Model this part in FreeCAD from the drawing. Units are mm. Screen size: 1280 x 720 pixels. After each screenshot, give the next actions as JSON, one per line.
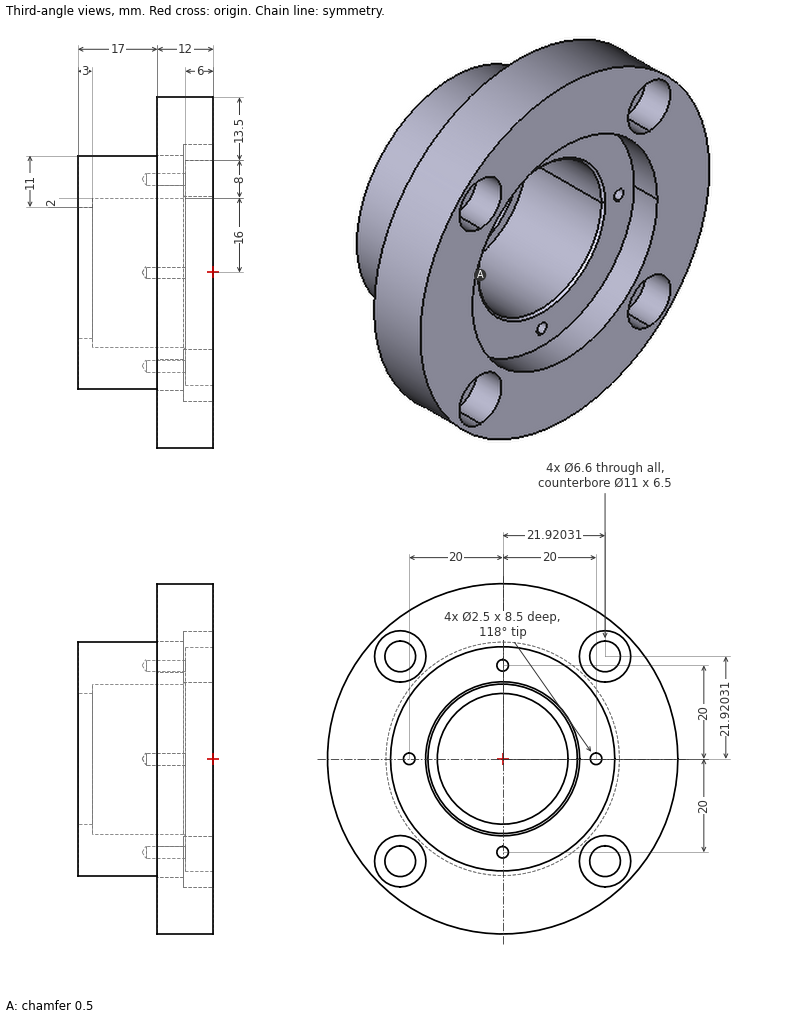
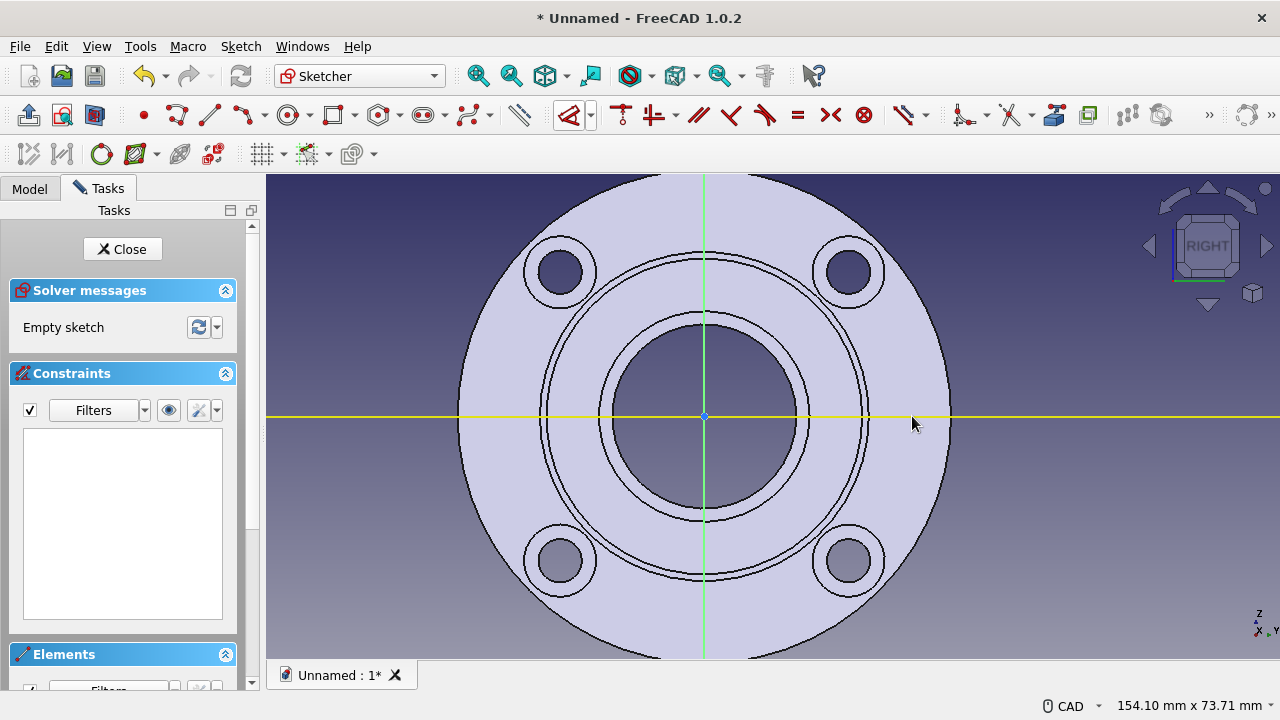
{"action": "key", "text": "g c"}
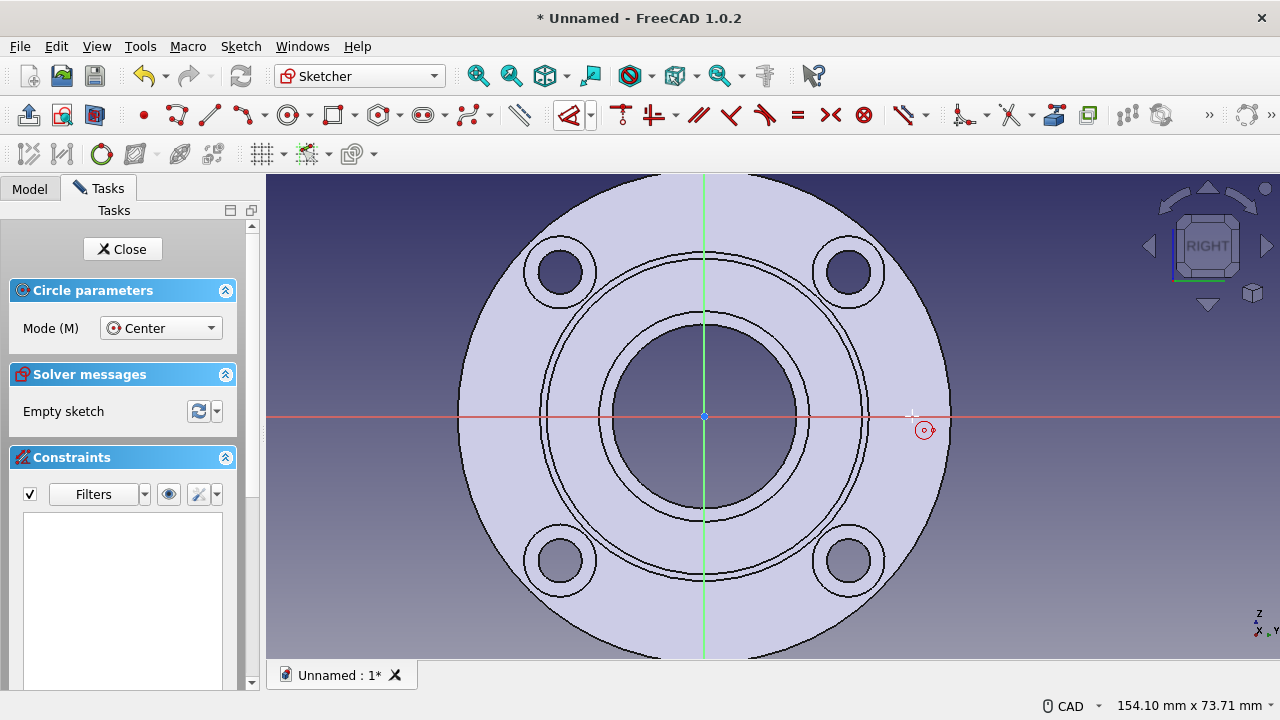
{"action": "scroll", "coordinate": [836, 416], "scroll_direction": "up", "scroll_amount": 6}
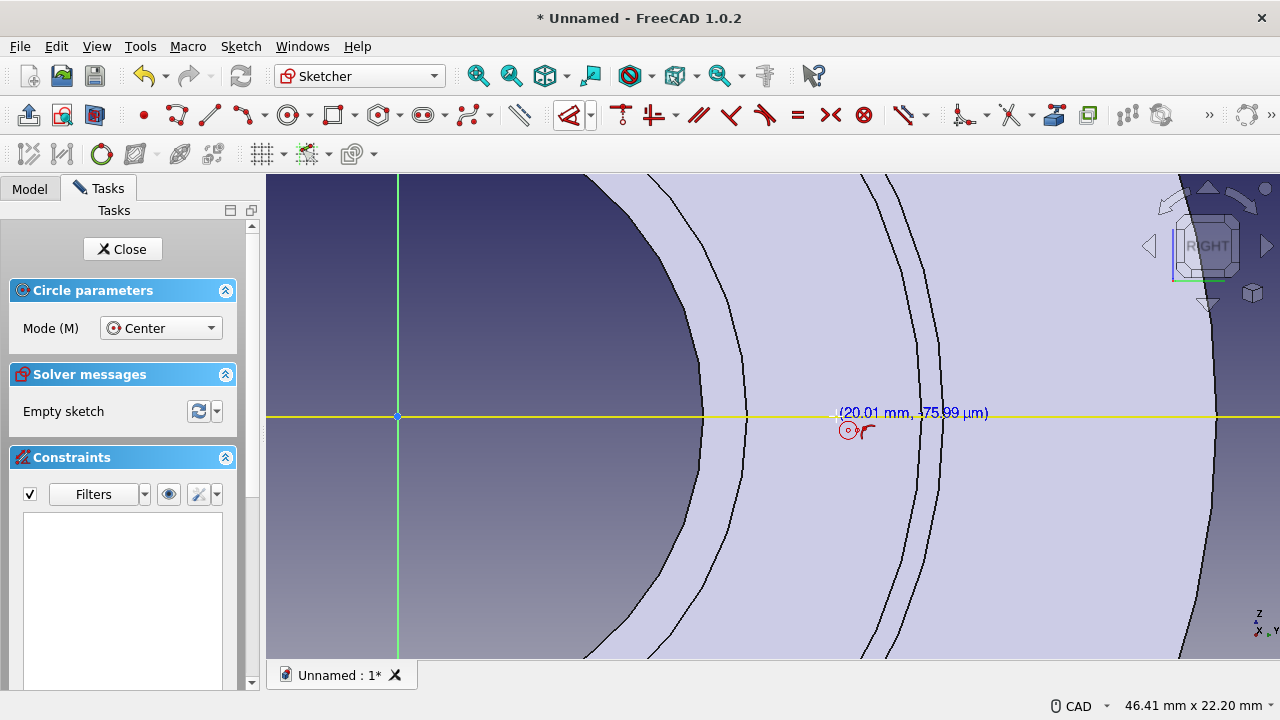
{"action": "left_click", "coordinate": [834, 416]}
{"action": "left_click", "coordinate": [854, 397]}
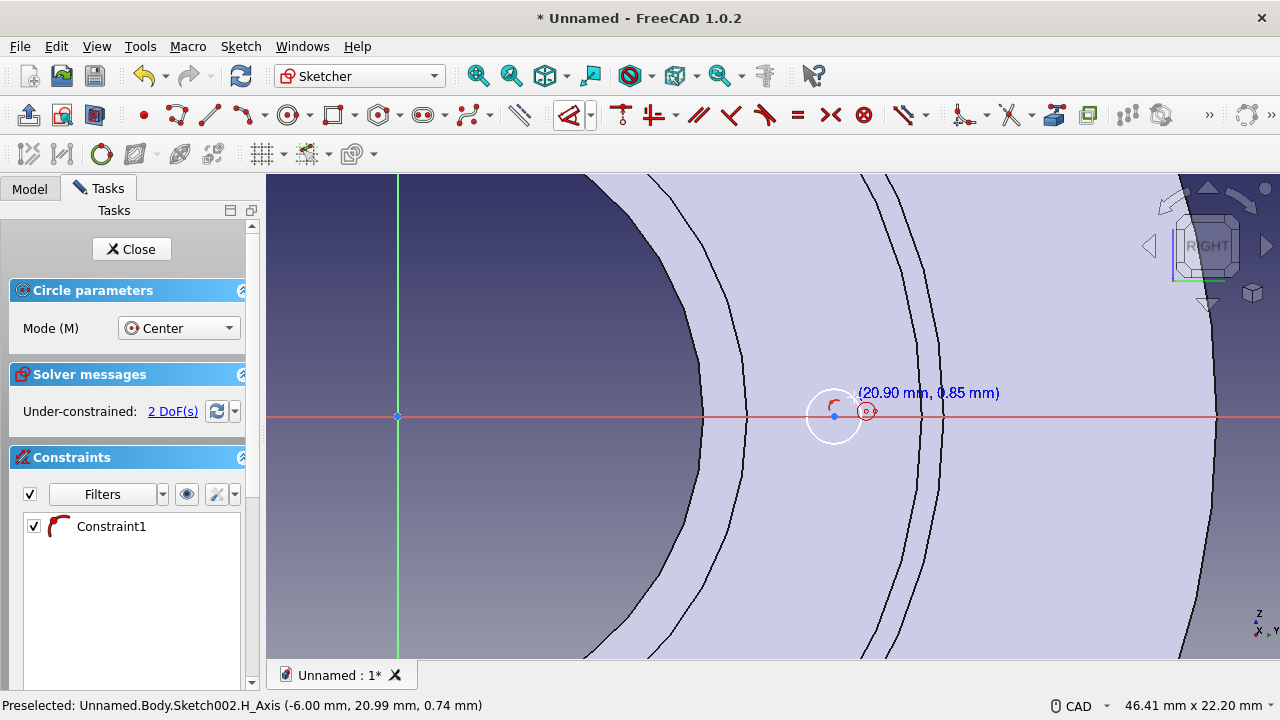
{"action": "scroll", "coordinate": [837, 416], "scroll_direction": "down", "scroll_amount": 6}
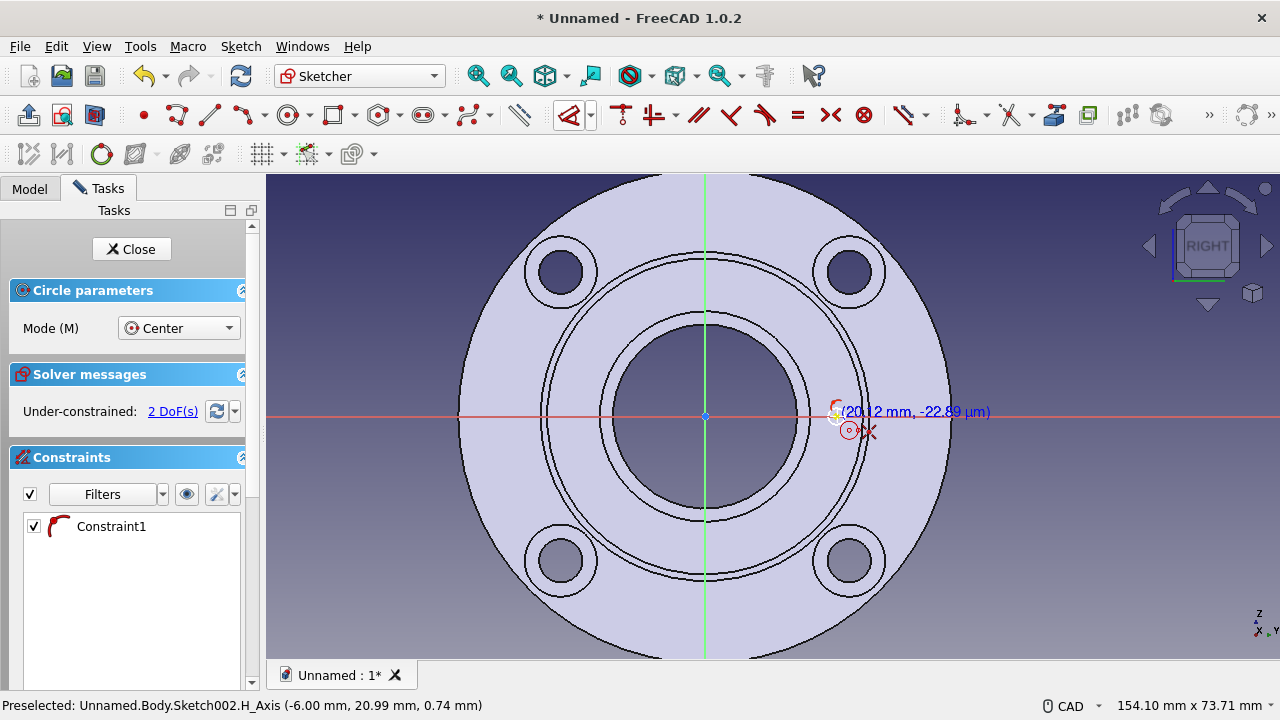
{"action": "scroll", "coordinate": [705, 285], "scroll_direction": "up", "scroll_amount": 6}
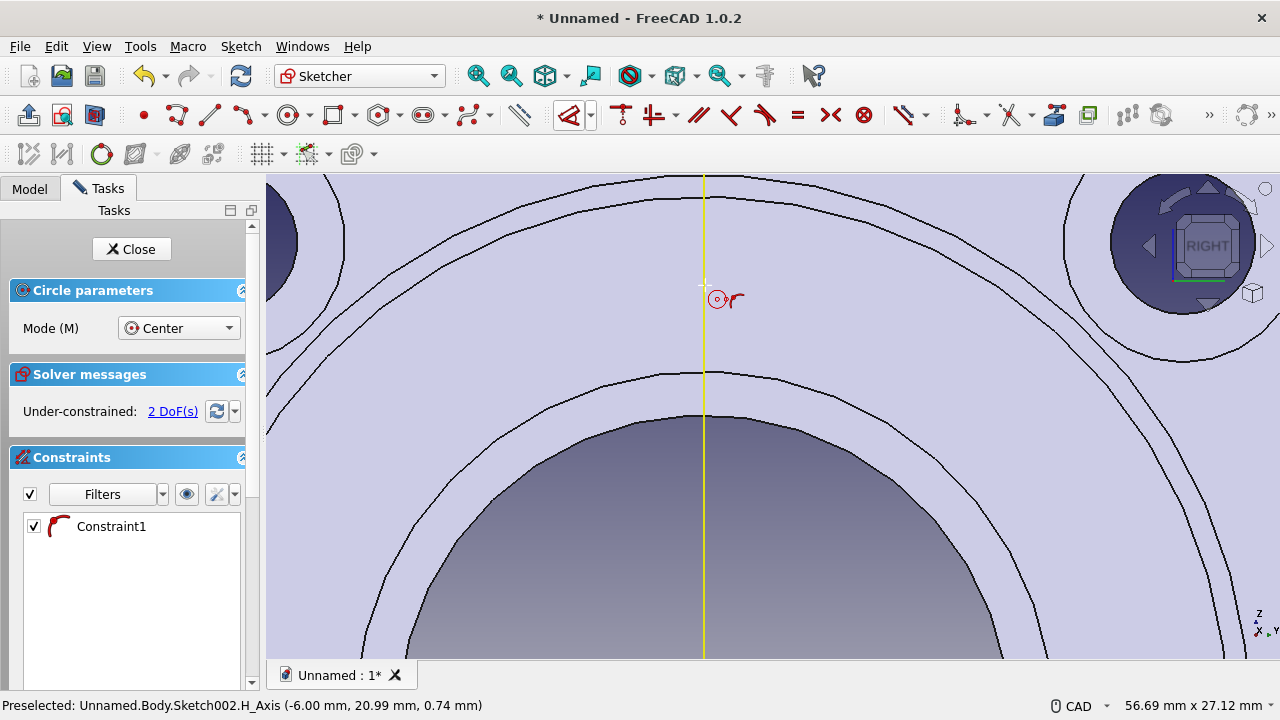
{"action": "left_click", "coordinate": [704, 284]}
{"action": "left_click", "coordinate": [723, 265]}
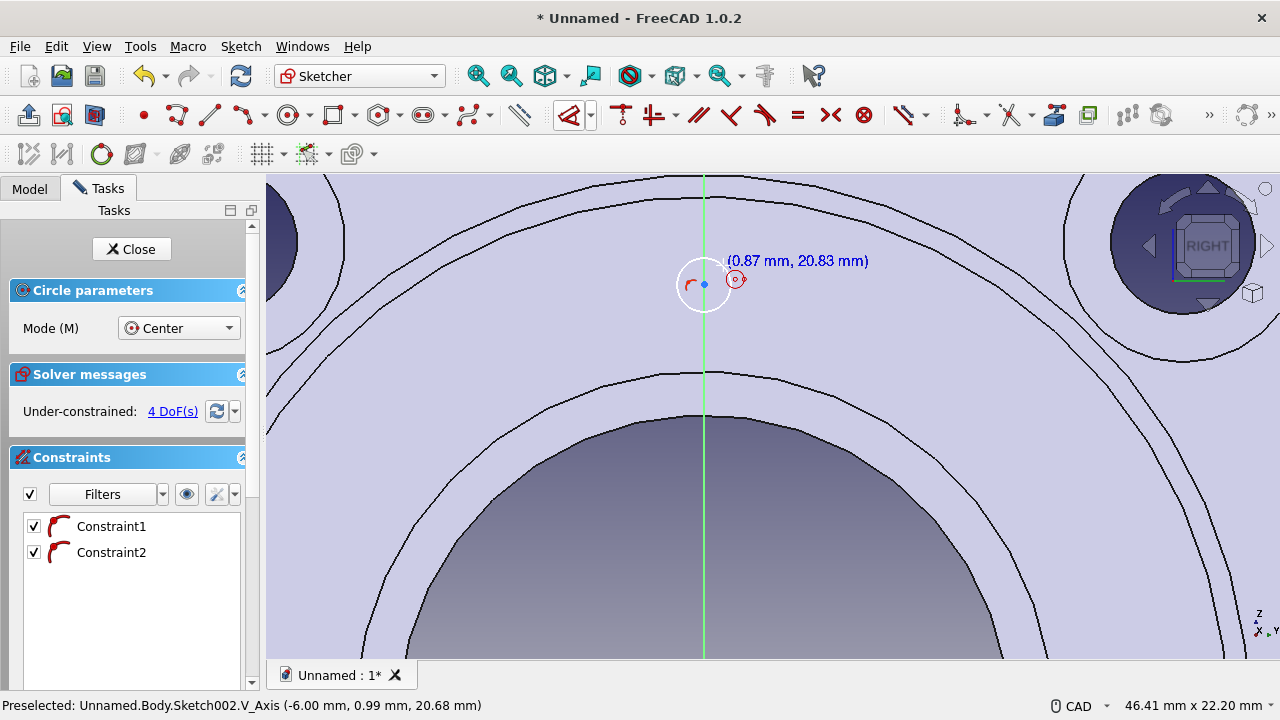
{"action": "scroll", "coordinate": [705, 285], "scroll_direction": "down", "scroll_amount": 6}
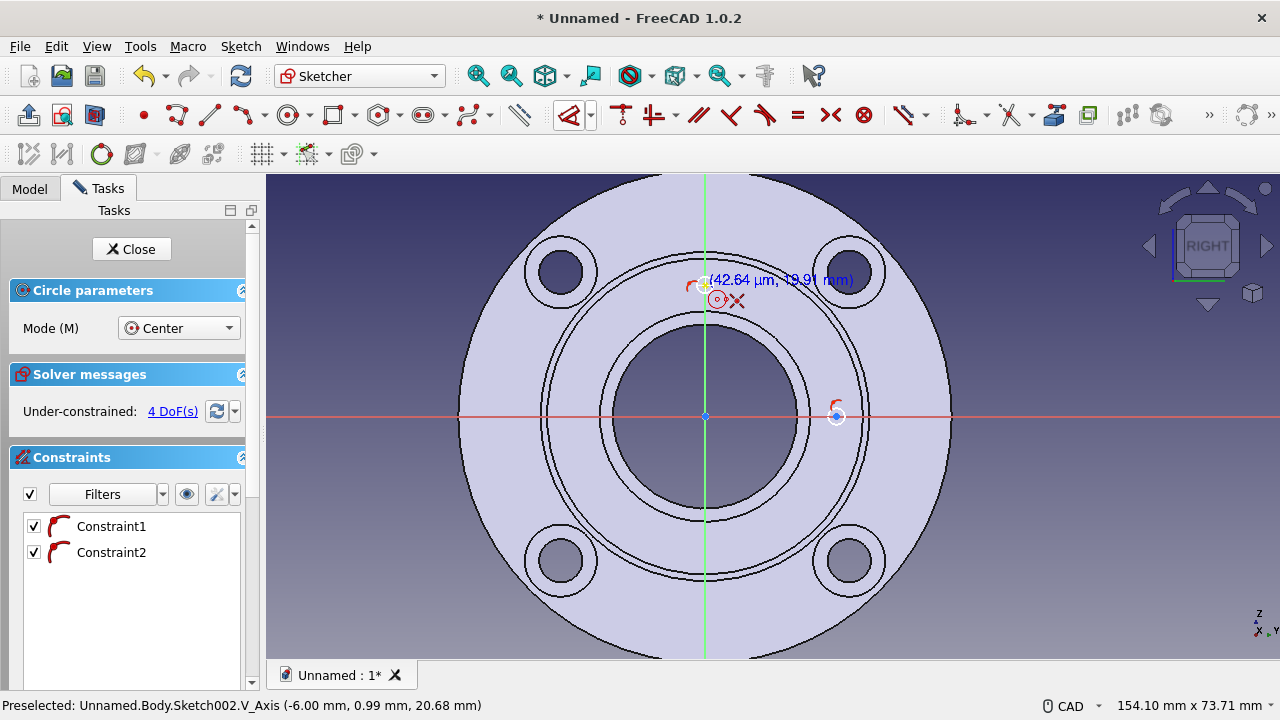
{"action": "scroll", "coordinate": [573, 416], "scroll_direction": "up", "scroll_amount": 6}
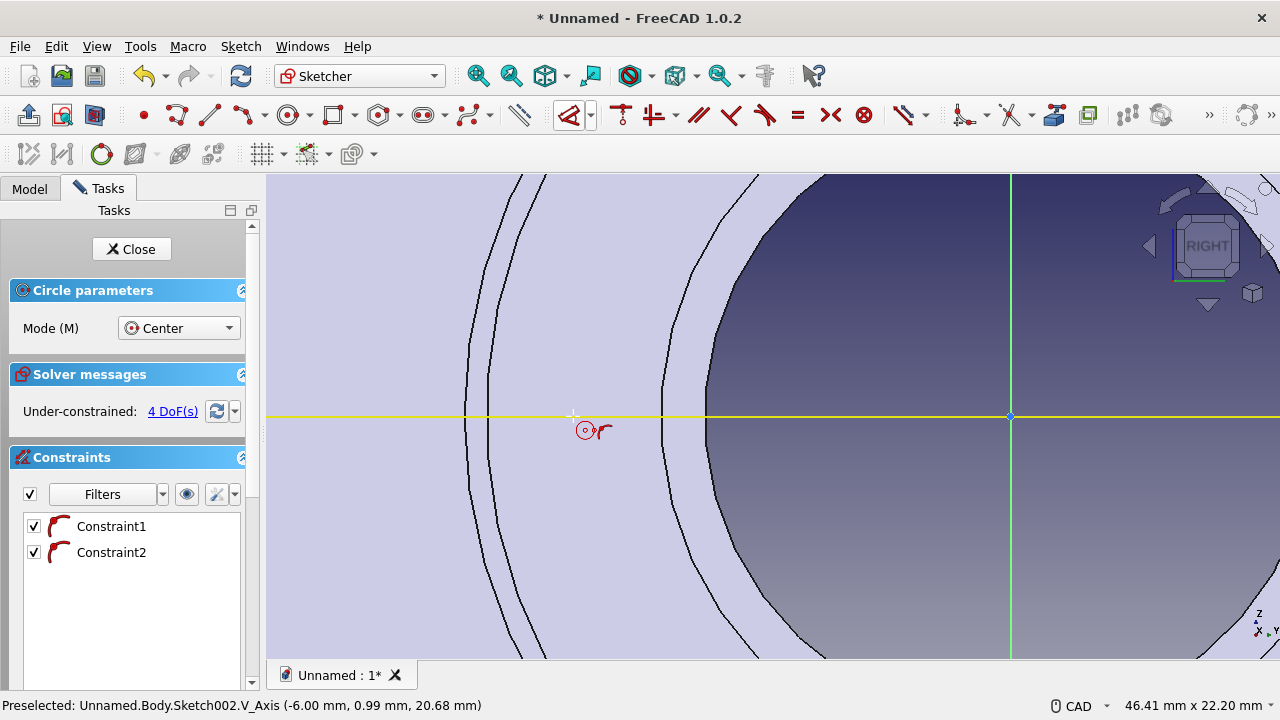
{"action": "left_click", "coordinate": [574, 416]}
{"action": "left_click", "coordinate": [593, 397]}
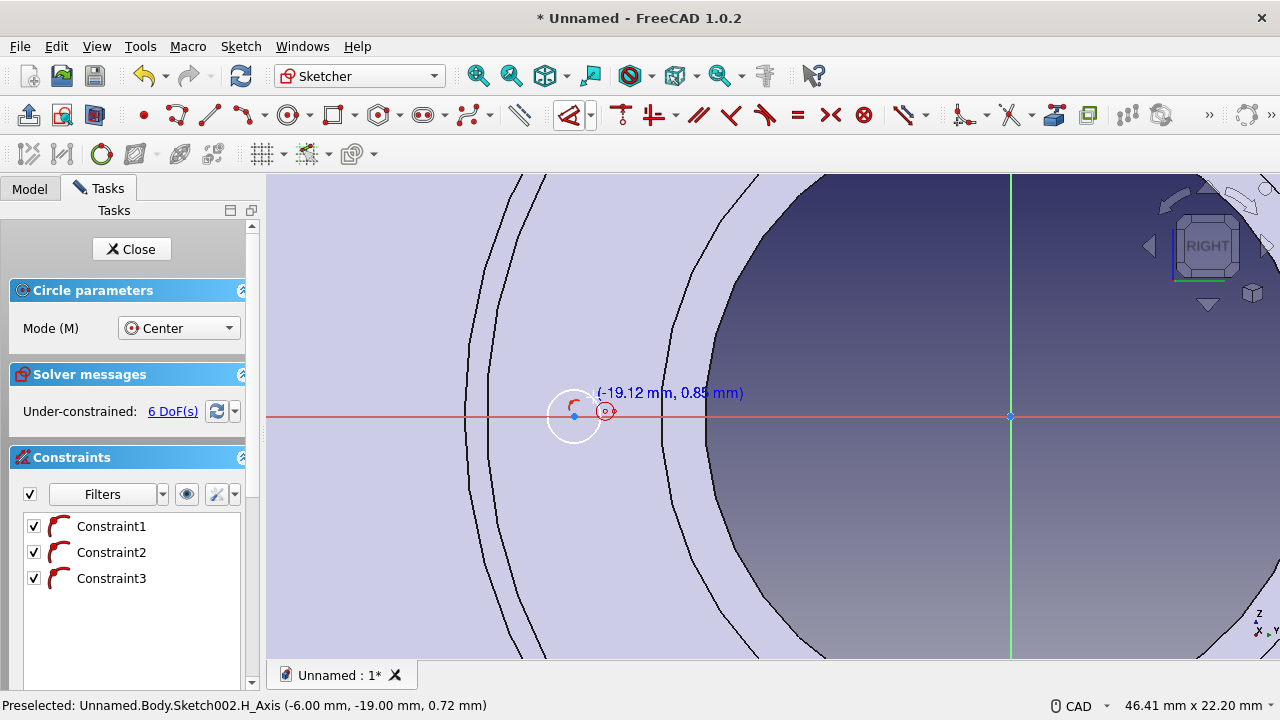
{"action": "scroll", "coordinate": [573, 416], "scroll_direction": "down", "scroll_amount": 6}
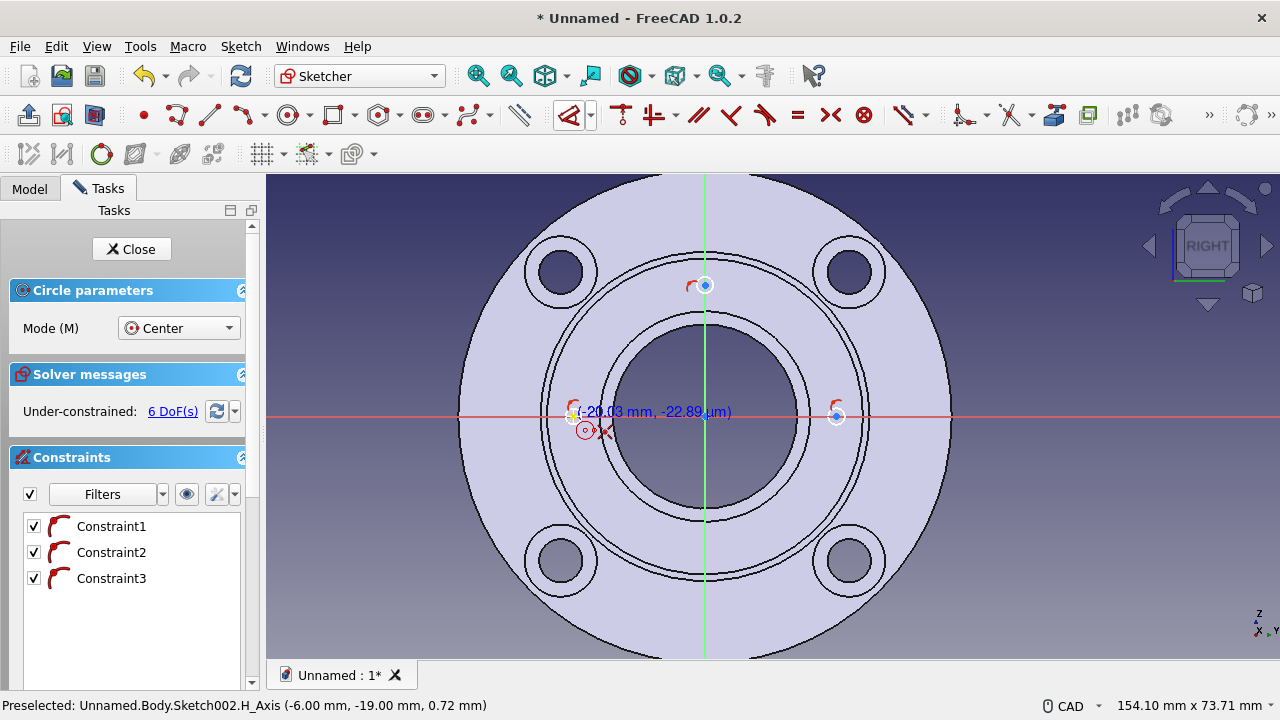
{"action": "scroll", "coordinate": [705, 548], "scroll_direction": "up", "scroll_amount": 6}